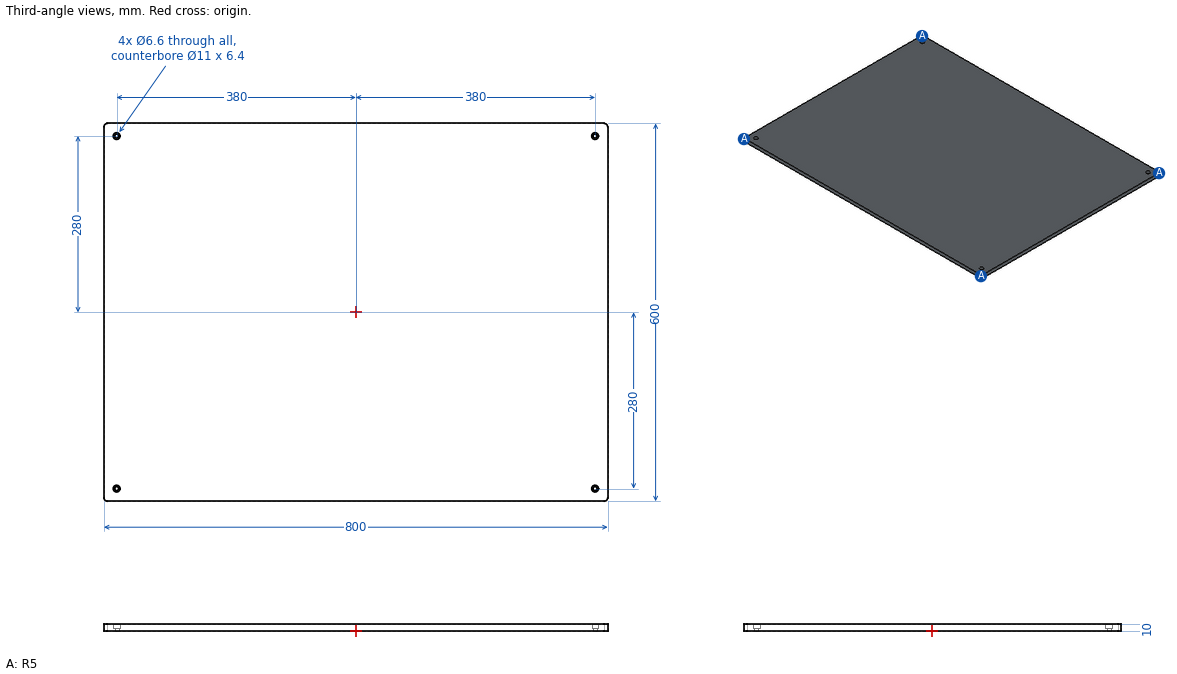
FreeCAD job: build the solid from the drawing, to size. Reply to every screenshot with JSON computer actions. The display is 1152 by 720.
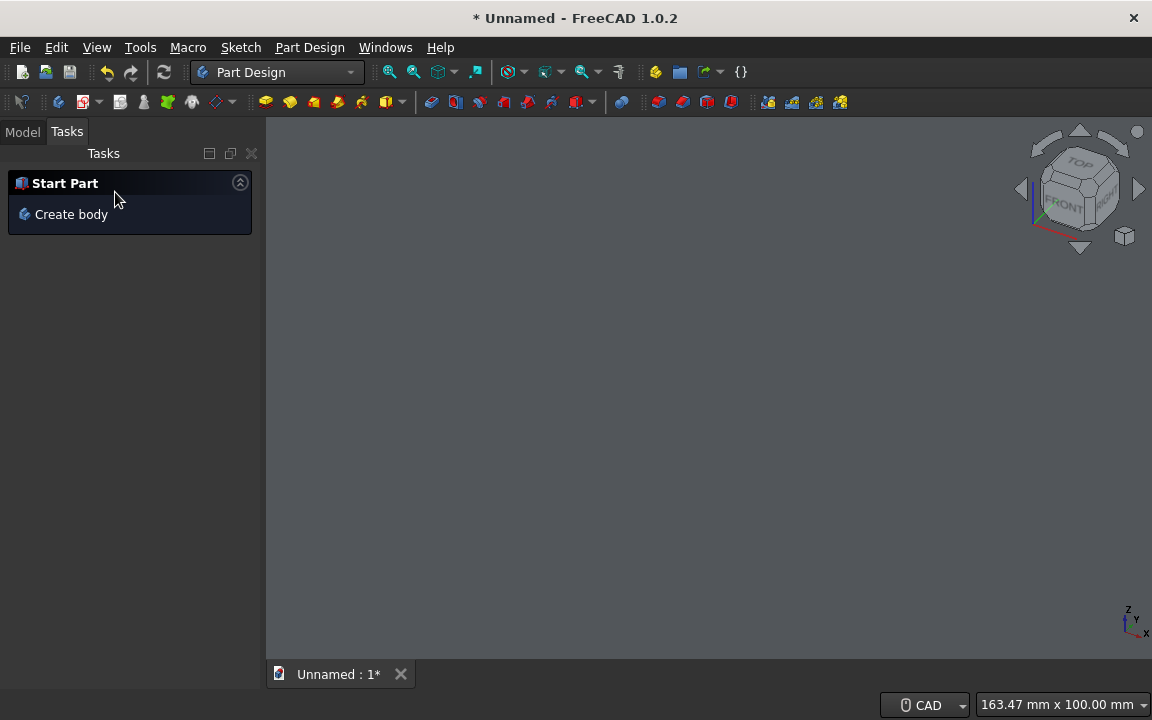
{"action": "key", "text": "v f"}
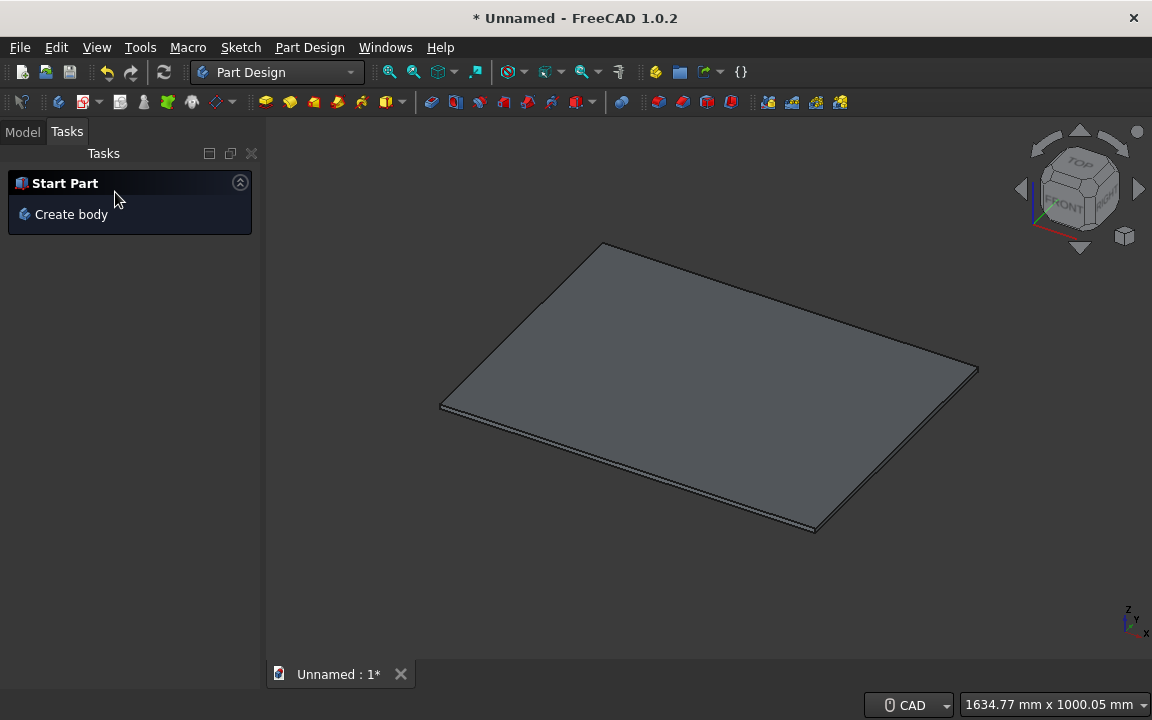
{"action": "left_click", "coordinate": [709, 385]}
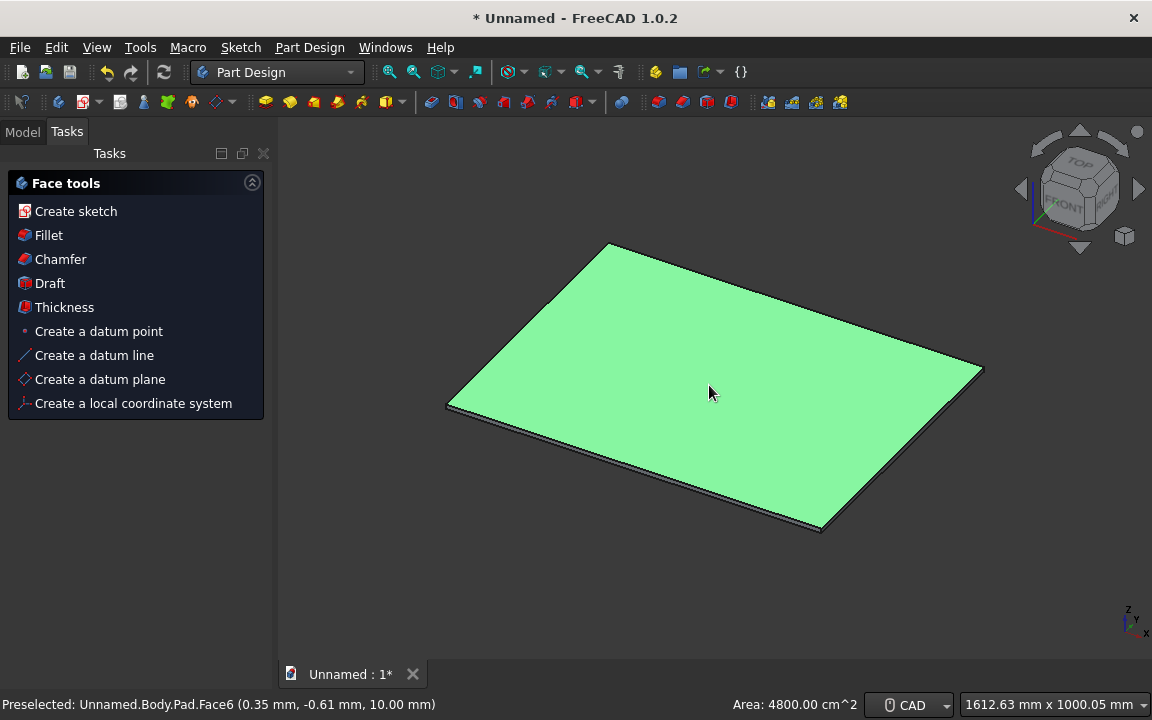
{"action": "left_click", "coordinate": [84, 102]}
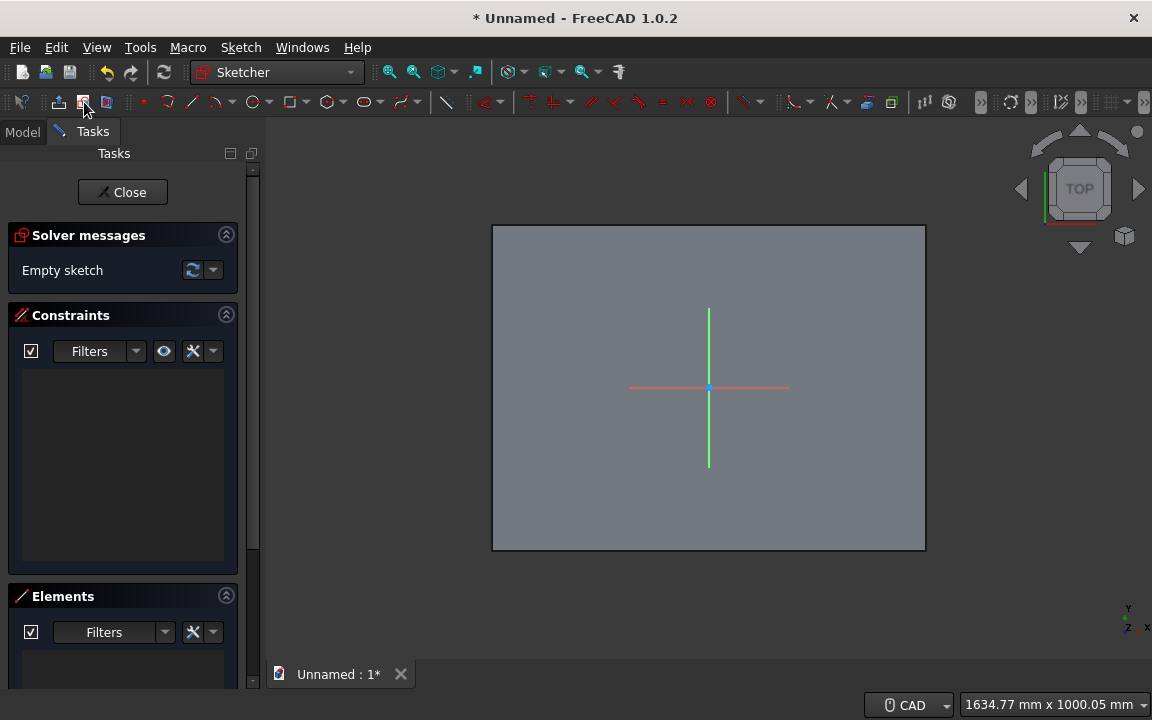
{"action": "left_click", "coordinate": [254, 102]}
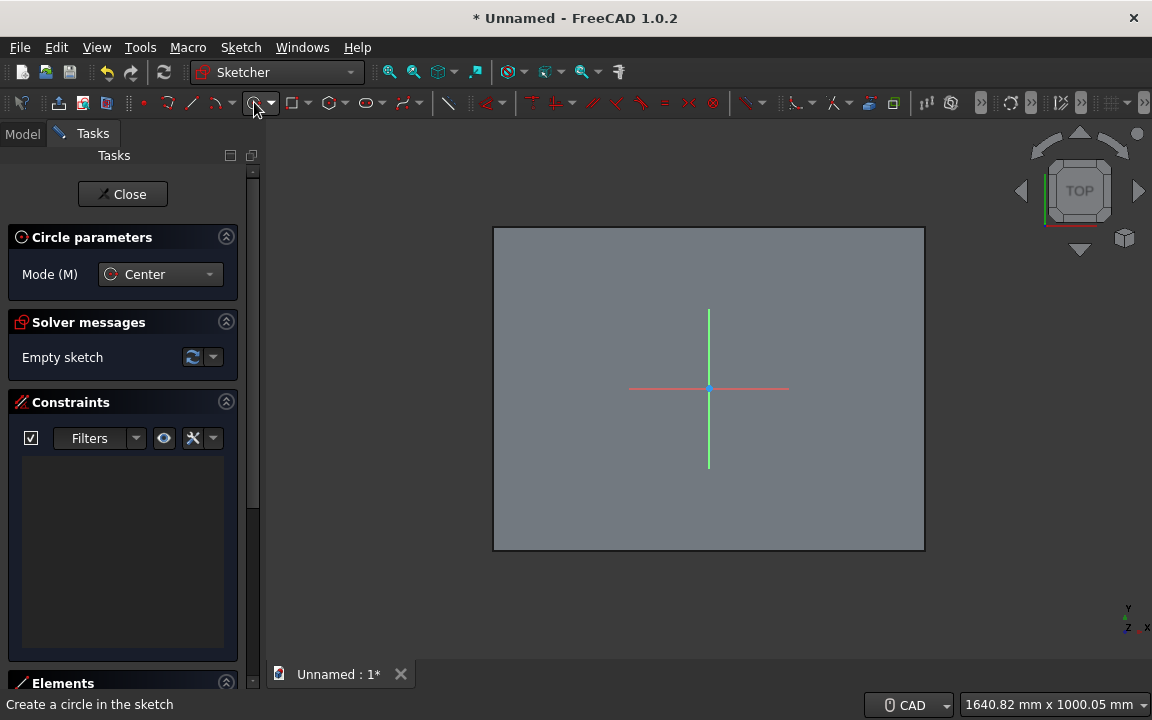
{"action": "scroll", "coordinate": [504, 238], "scroll_direction": "up", "scroll_amount": 13}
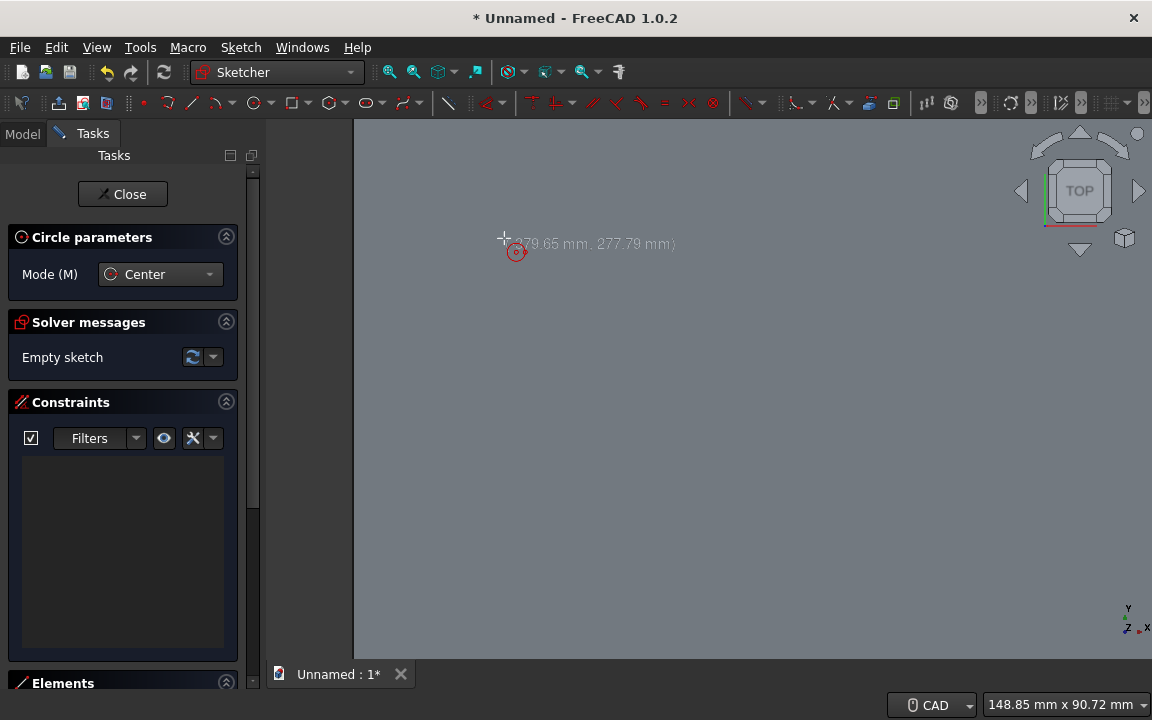
{"action": "scroll", "coordinate": [379, 202], "scroll_direction": "down", "scroll_amount": 12}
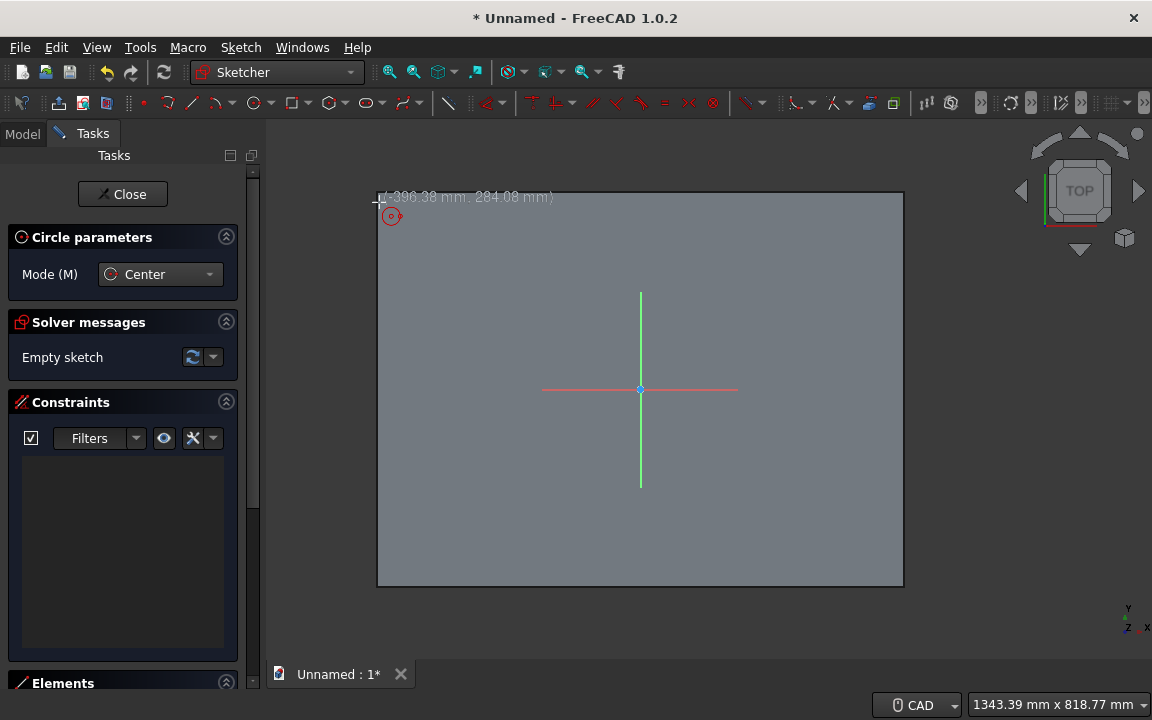
{"action": "left_click", "coordinate": [390, 205]}
{"action": "mouse_move", "coordinate": [391, 203]}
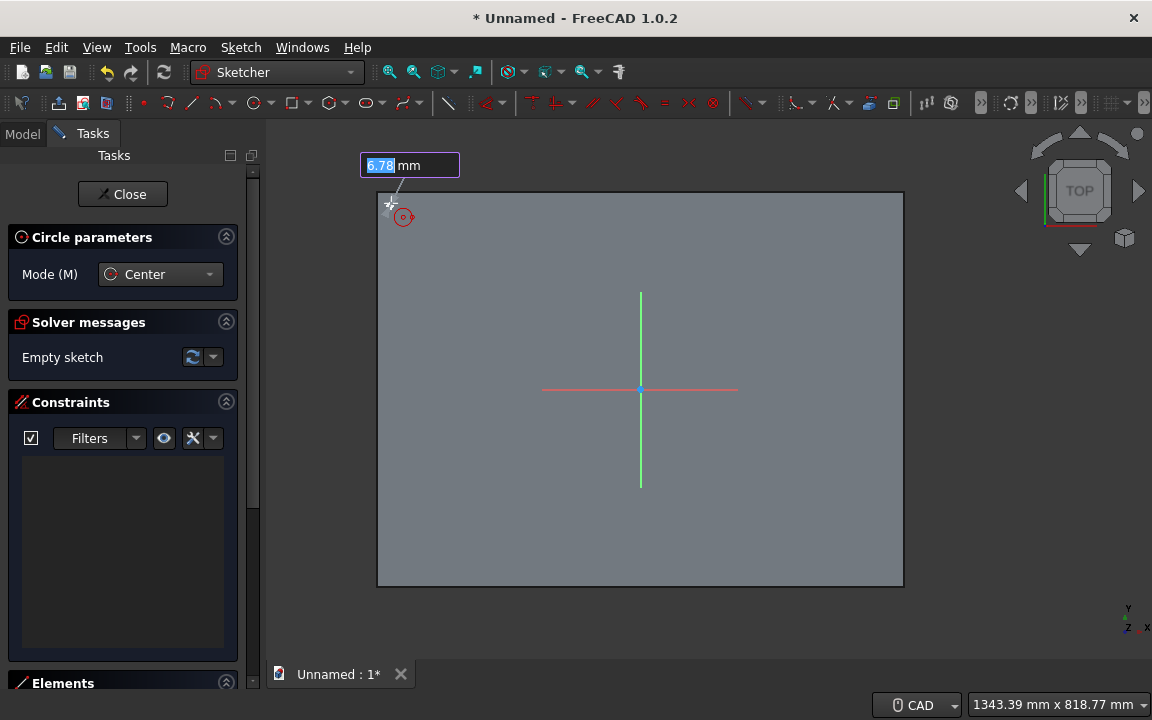
{"action": "type", "text": "6.6"}
{"action": "key", "text": "Return"}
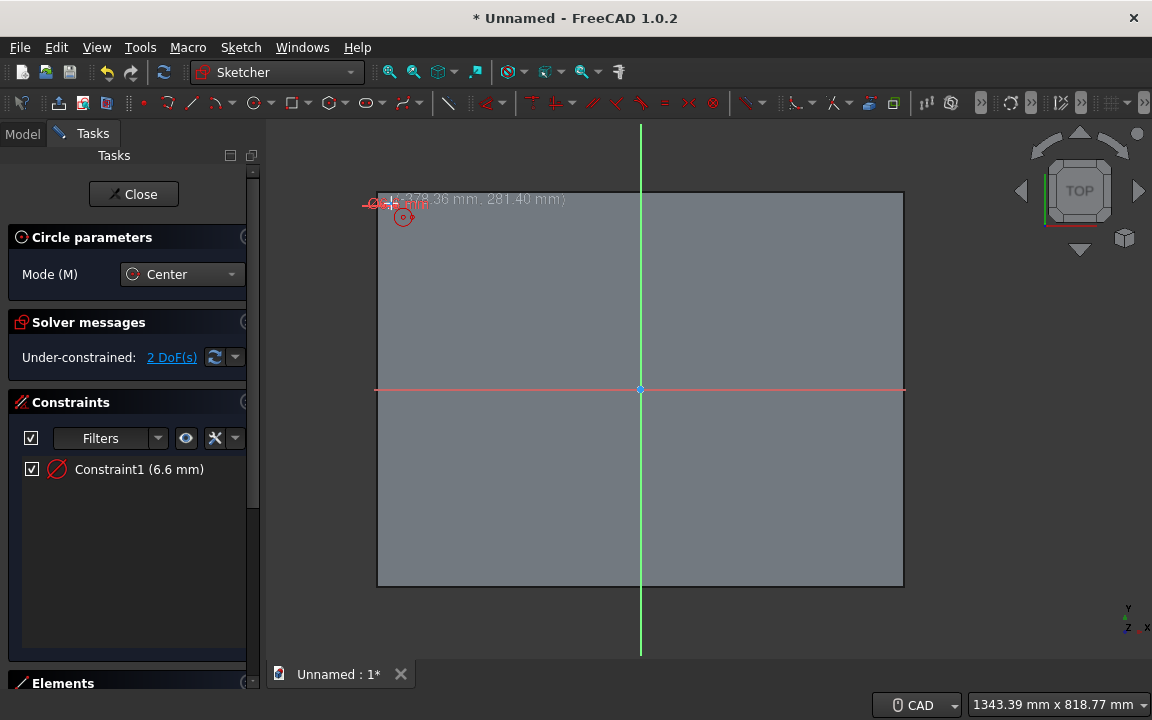
{"action": "scroll", "coordinate": [891, 205], "scroll_direction": "up", "scroll_amount": 12}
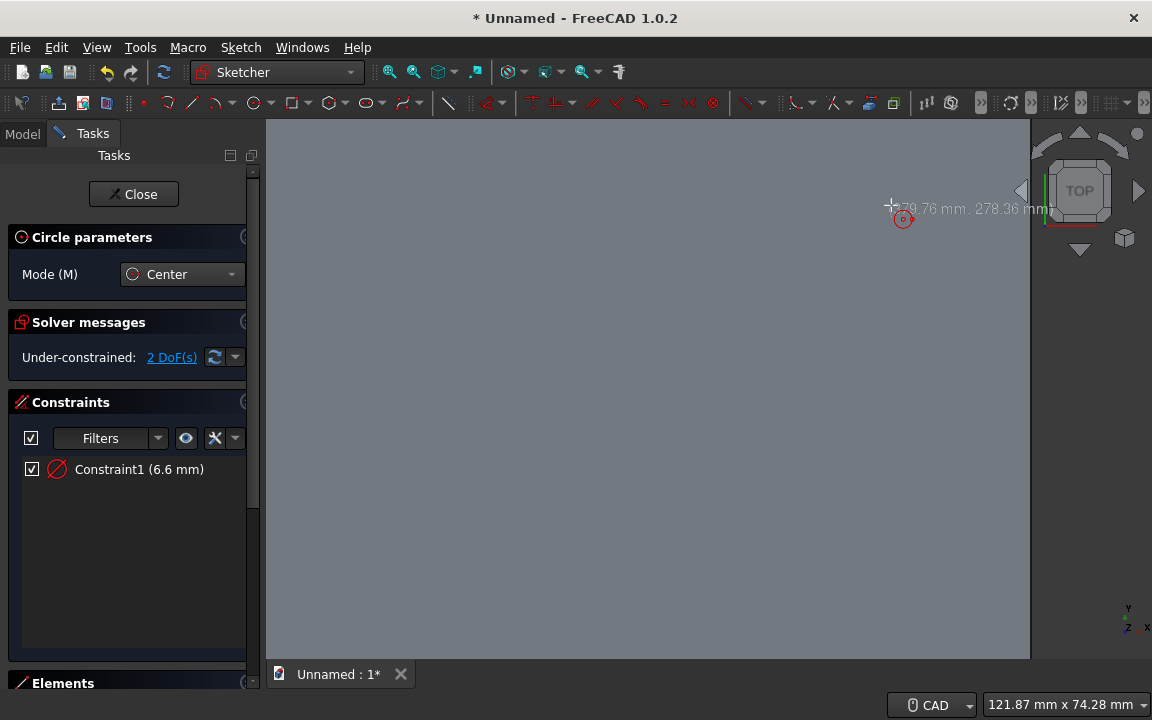
{"action": "scroll", "coordinate": [892, 205], "scroll_direction": "down", "scroll_amount": 12}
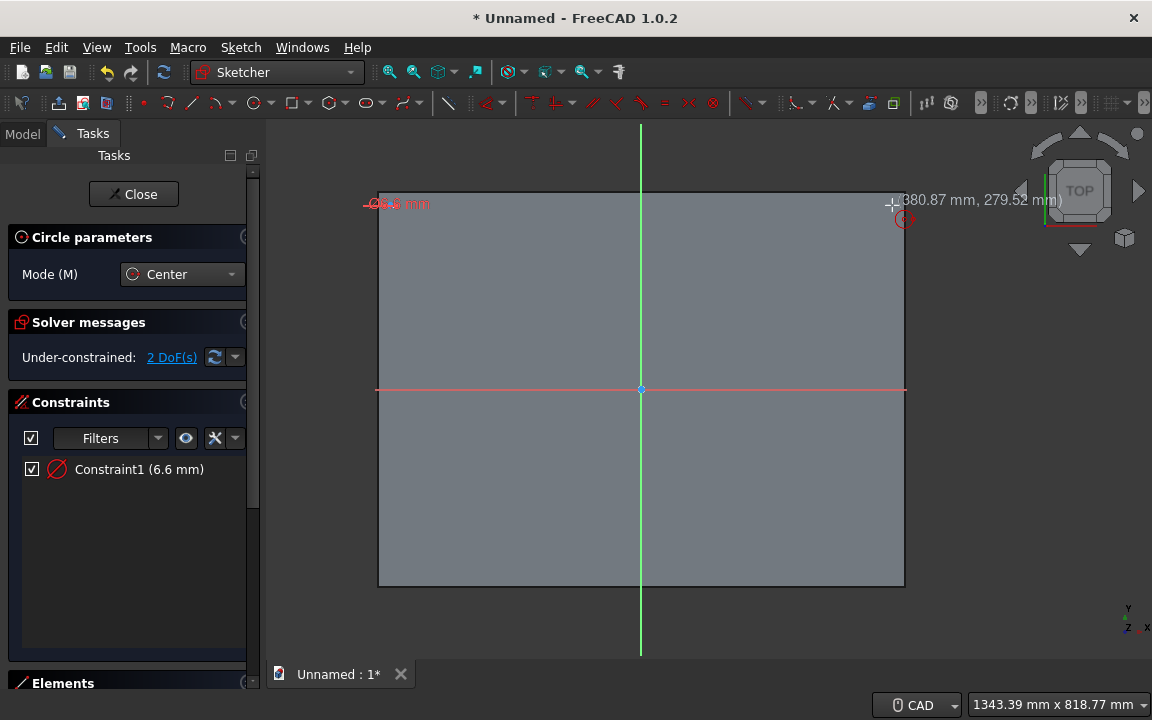
{"action": "left_click", "coordinate": [892, 205]}
{"action": "mouse_move", "coordinate": [894, 203]}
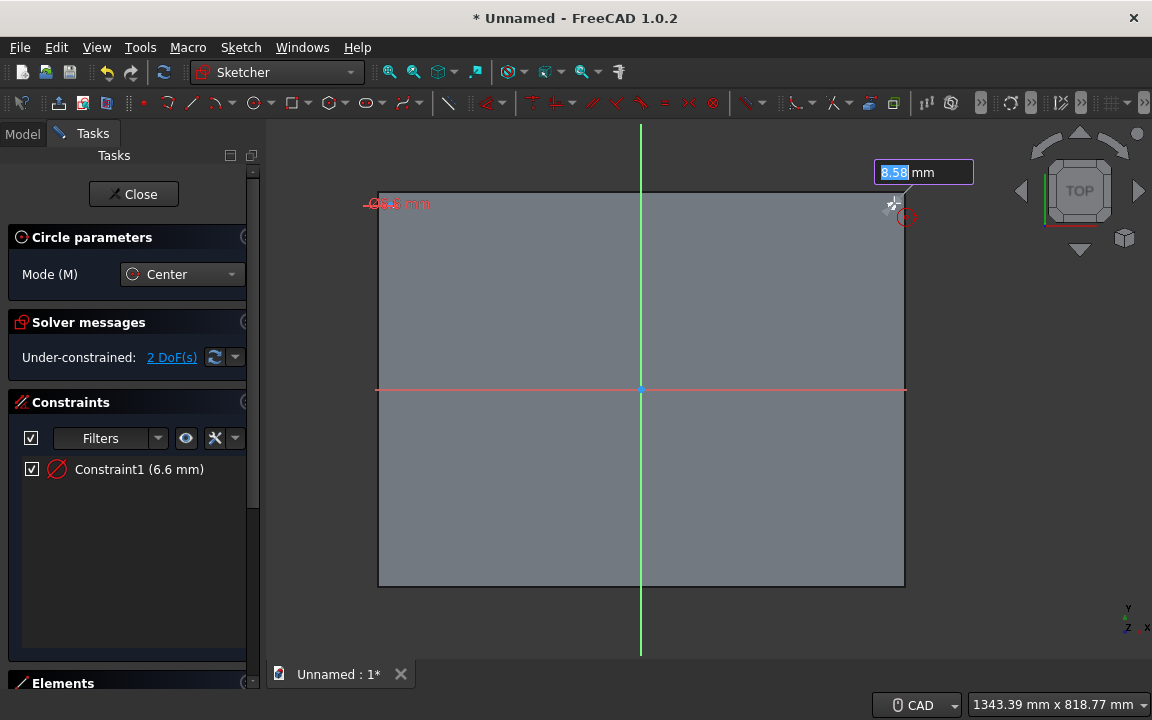
{"action": "type", "text": "6.6"}
{"action": "key", "text": "Return"}